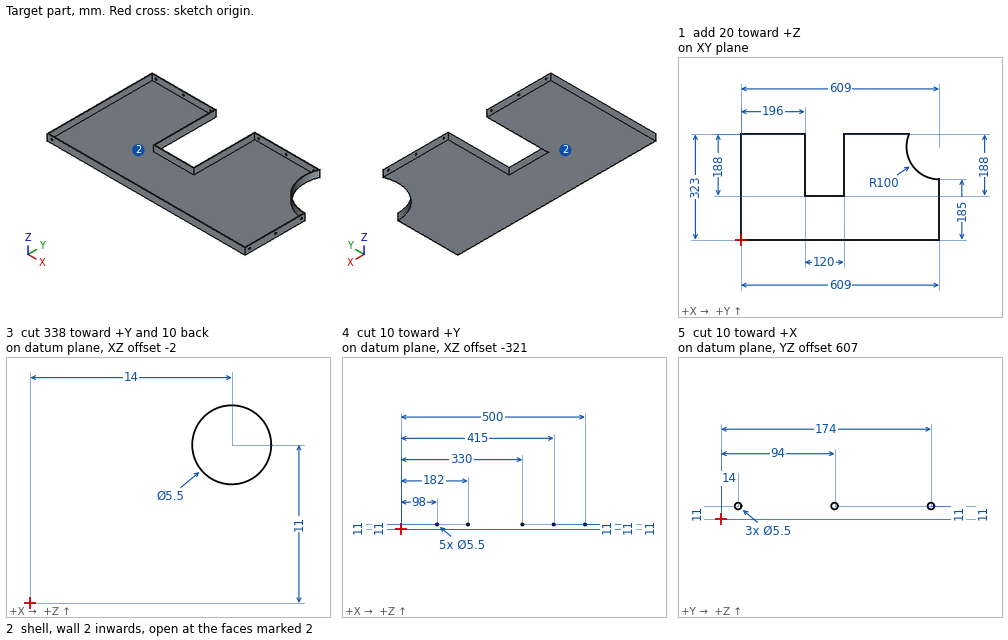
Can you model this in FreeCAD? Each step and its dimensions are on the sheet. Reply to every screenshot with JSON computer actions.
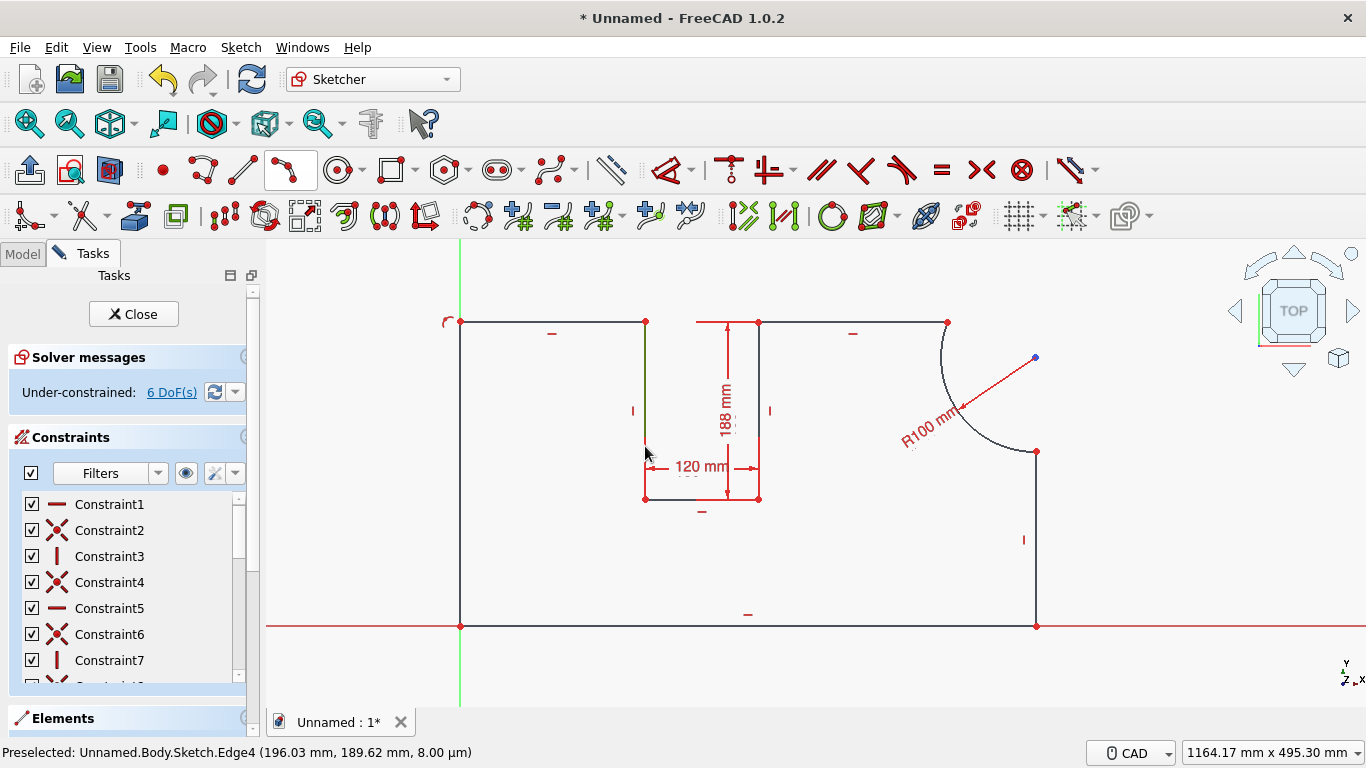
{"action": "key", "text": "i"}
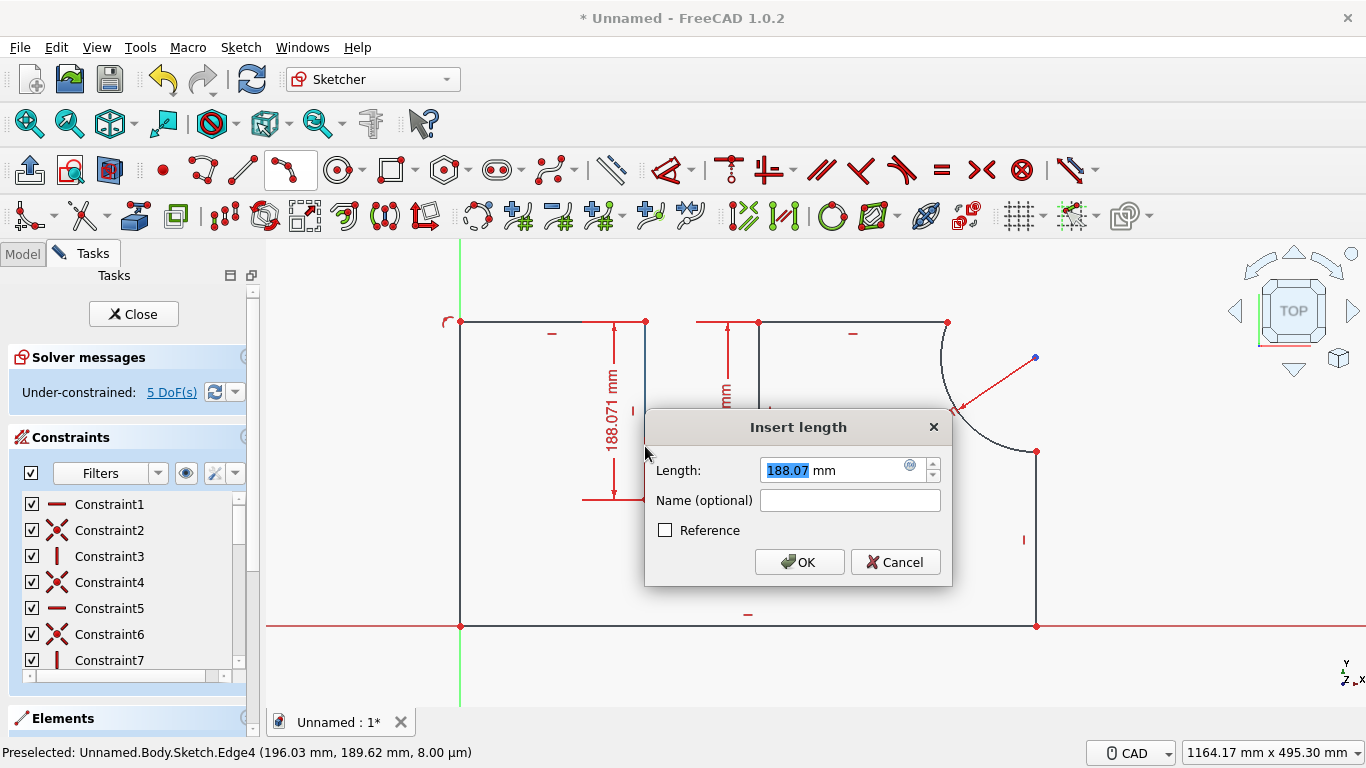
{"action": "type", "text": "188"}
{"action": "key", "text": "Return"}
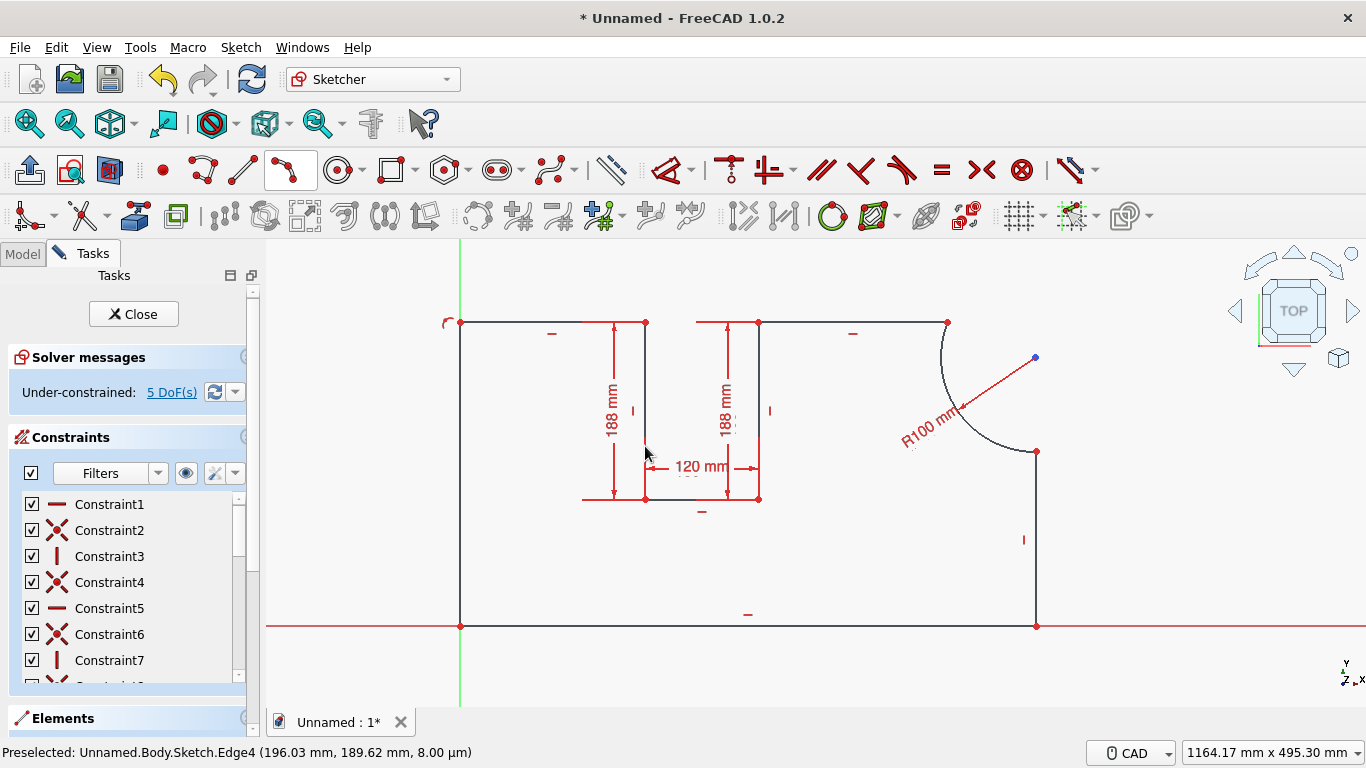
{"action": "left_click", "coordinate": [590, 322]}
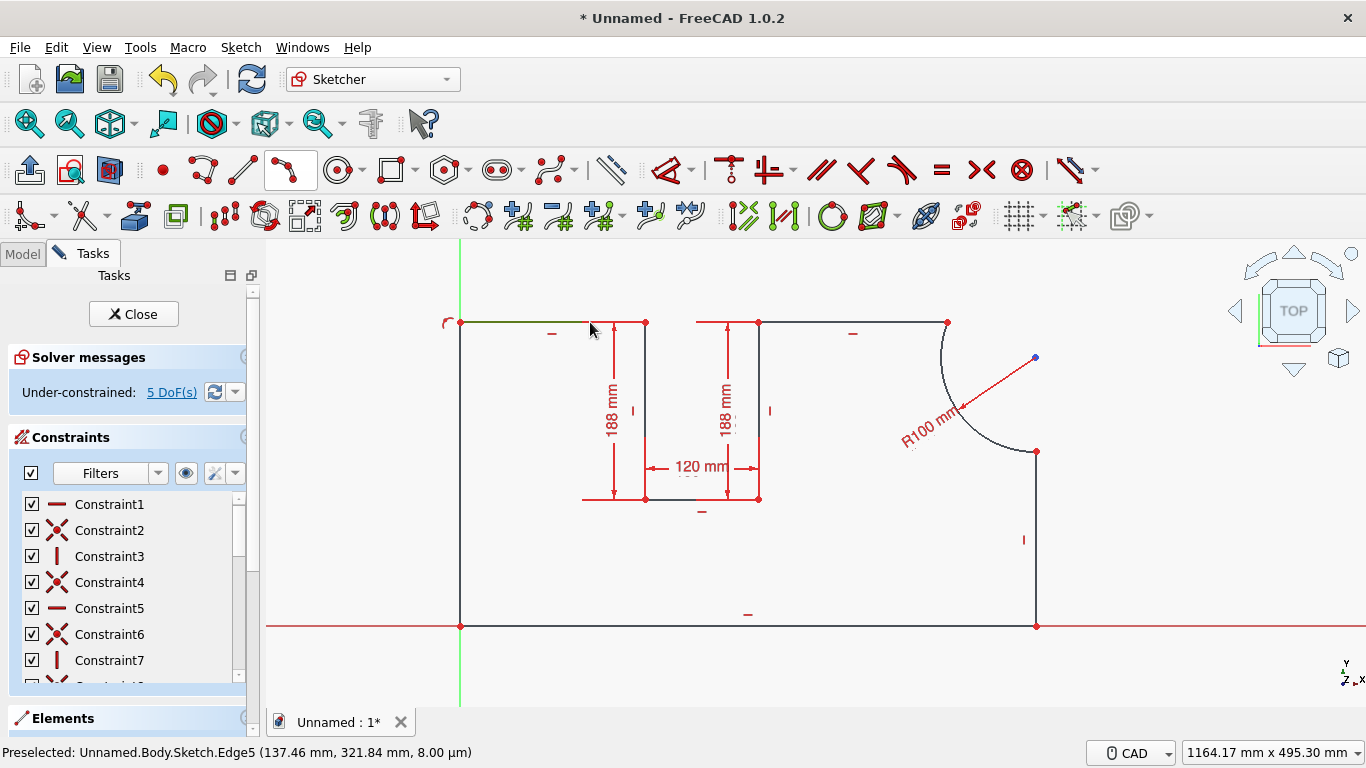
{"action": "key", "text": "l"}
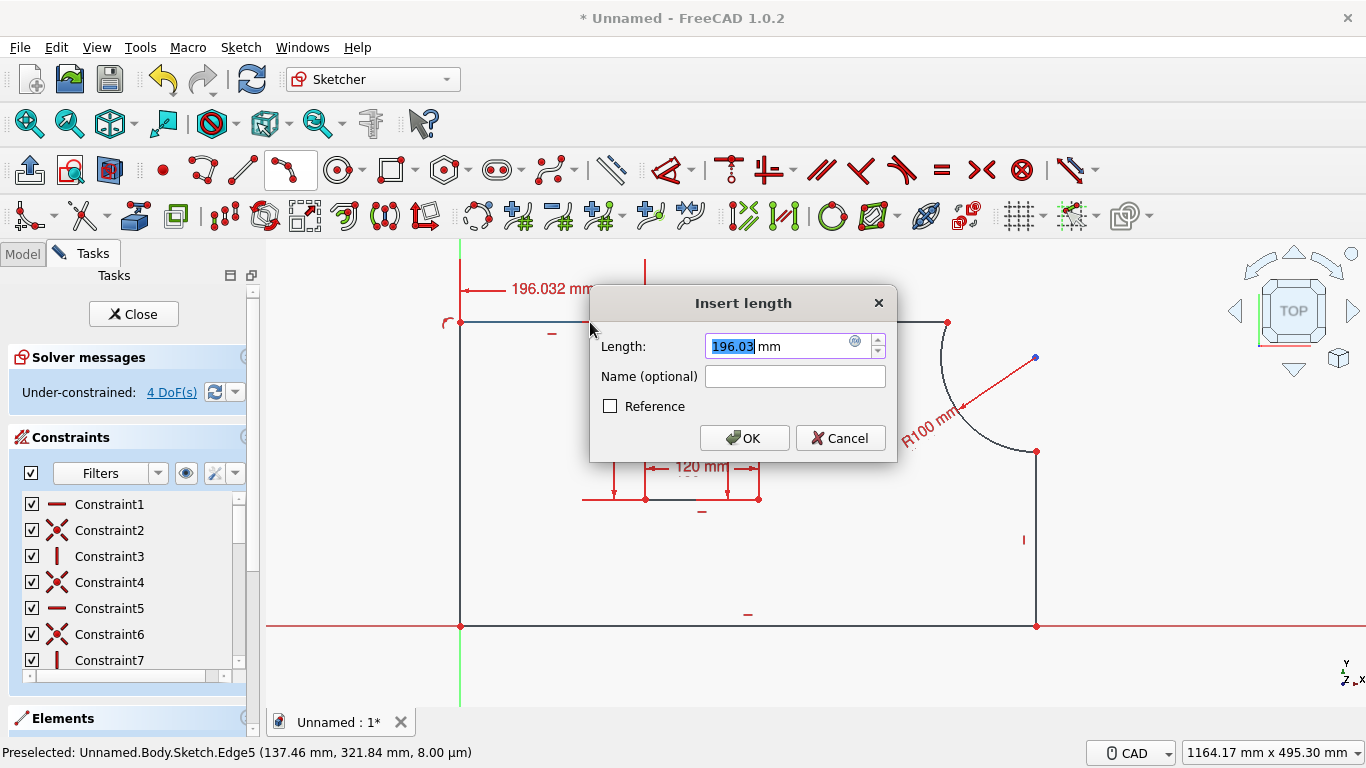
{"action": "type", "text": "196"}
{"action": "key", "text": "Return"}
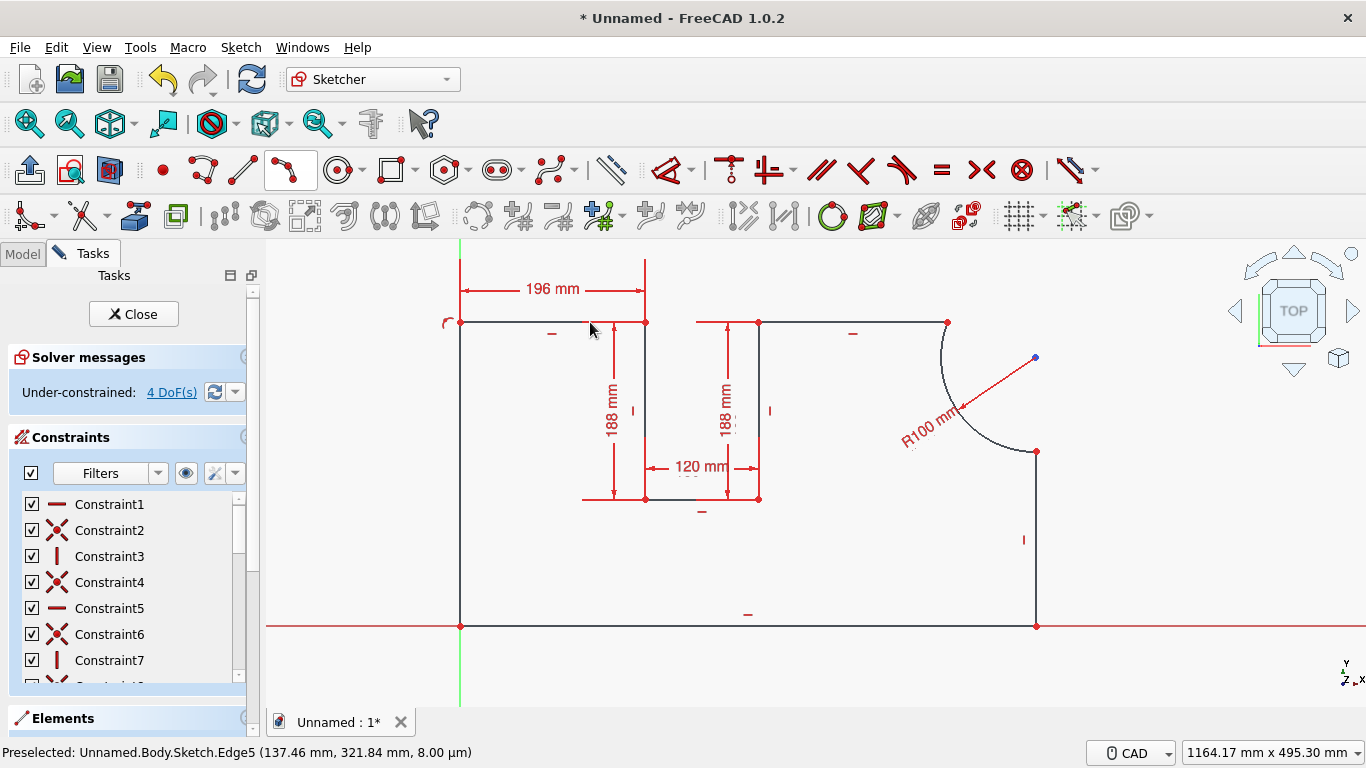
{"action": "left_click", "coordinate": [460, 413]}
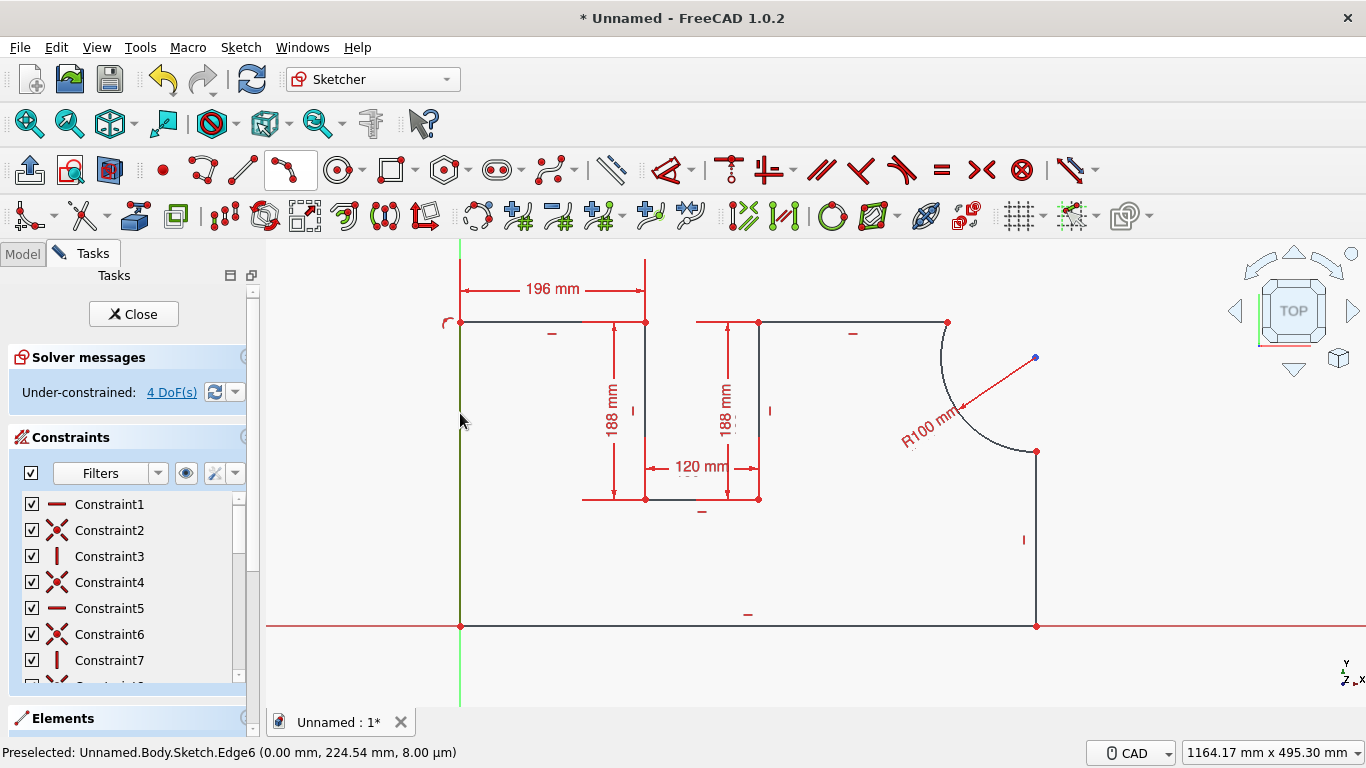
{"action": "key", "text": "i"}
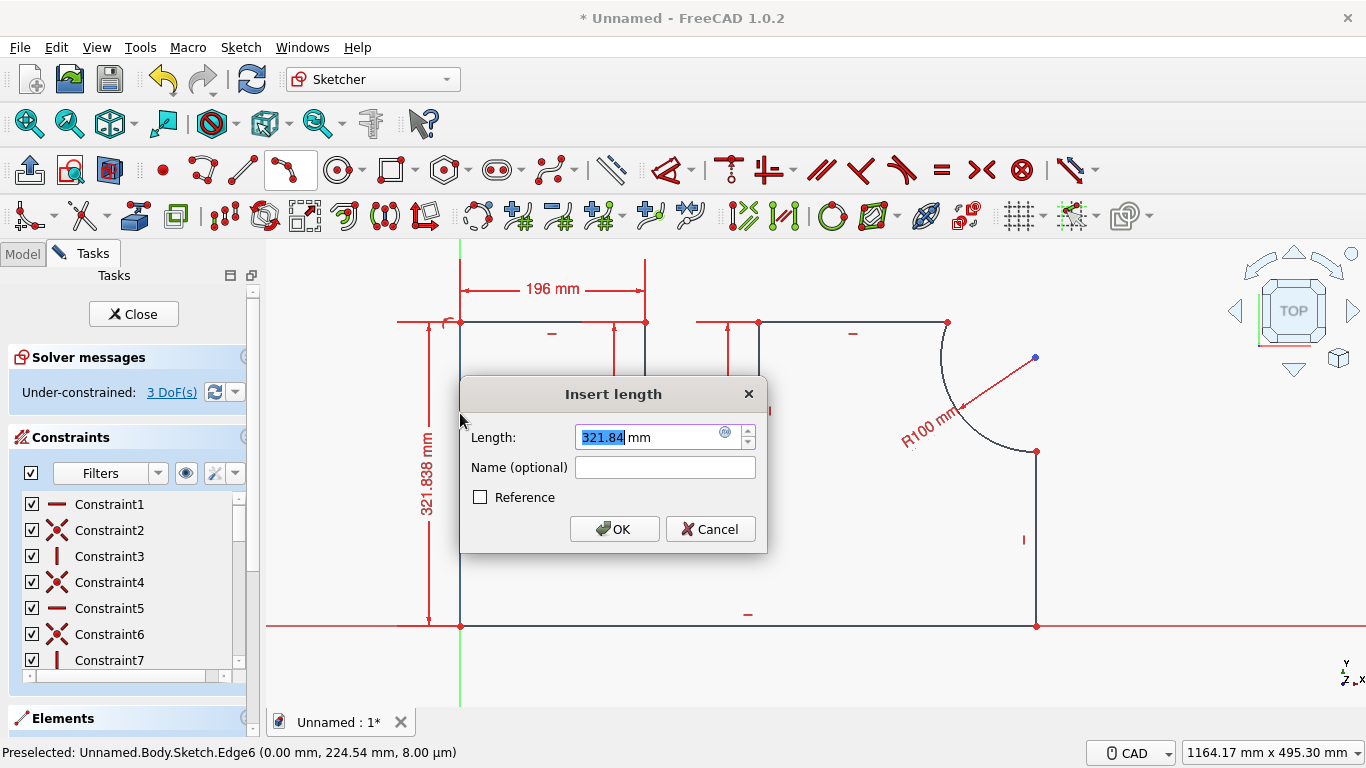
{"action": "type", "text": "323"}
{"action": "key", "text": "Return"}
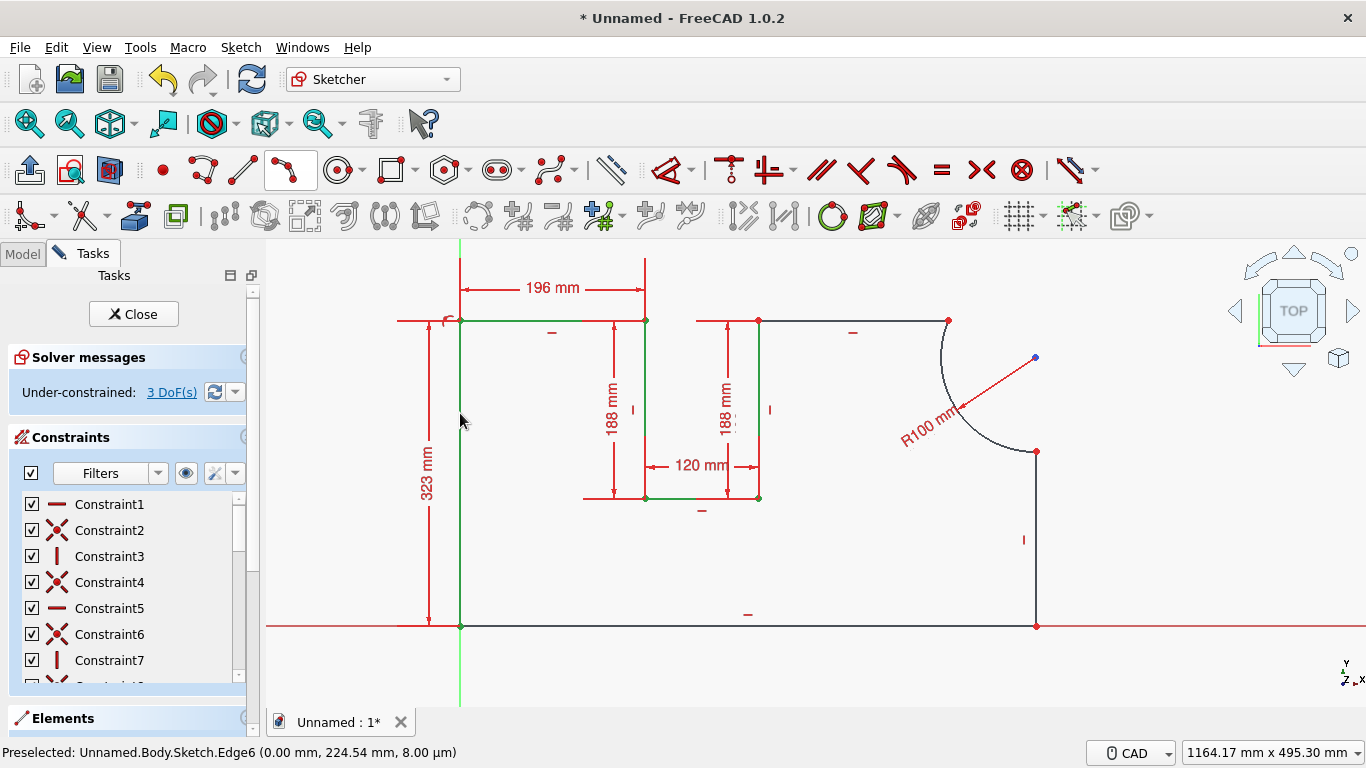
{"action": "left_click", "coordinate": [633, 626]}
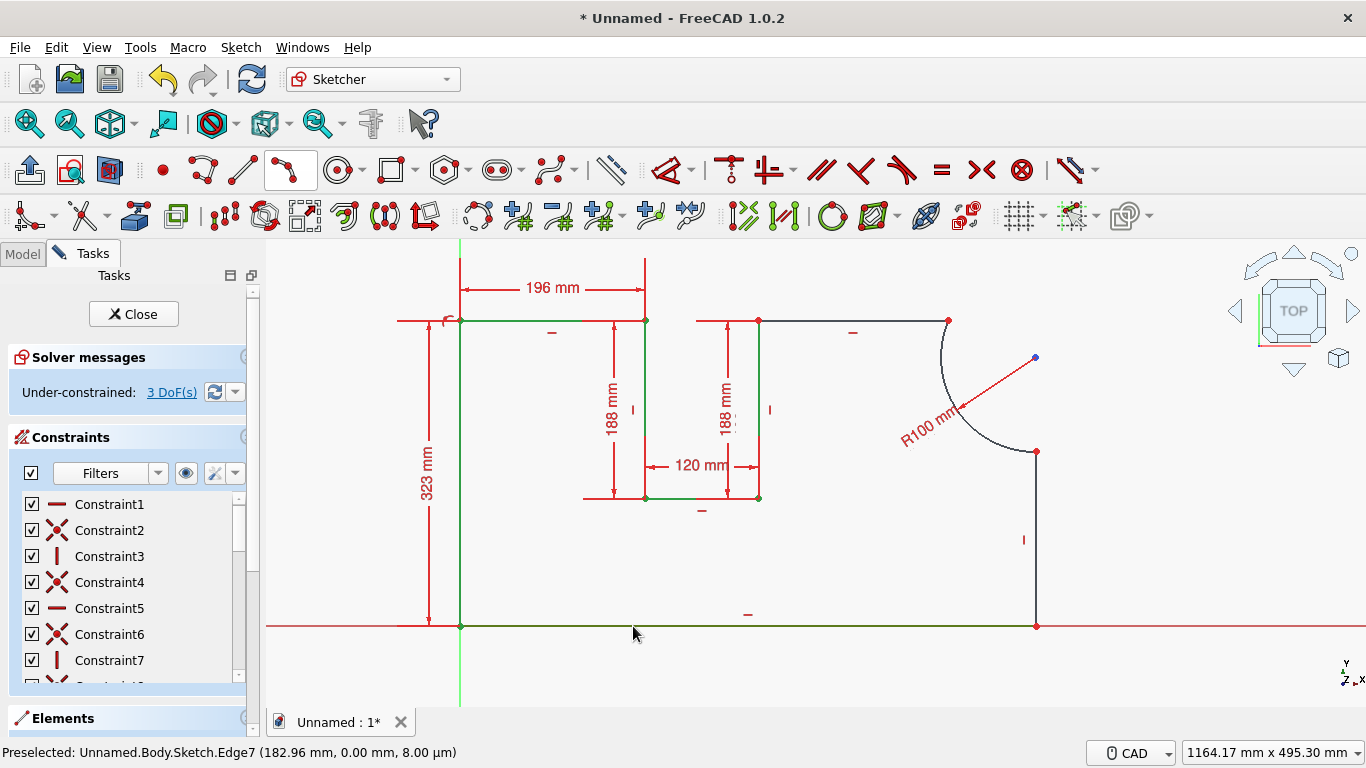
{"action": "key", "text": "l"}